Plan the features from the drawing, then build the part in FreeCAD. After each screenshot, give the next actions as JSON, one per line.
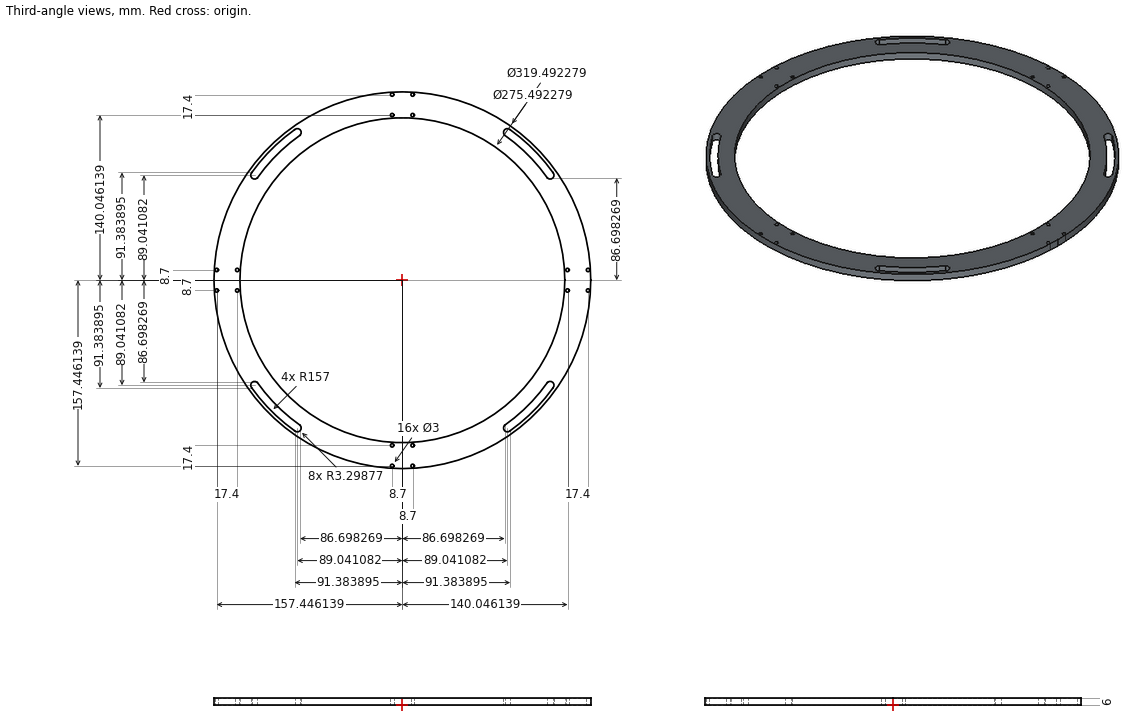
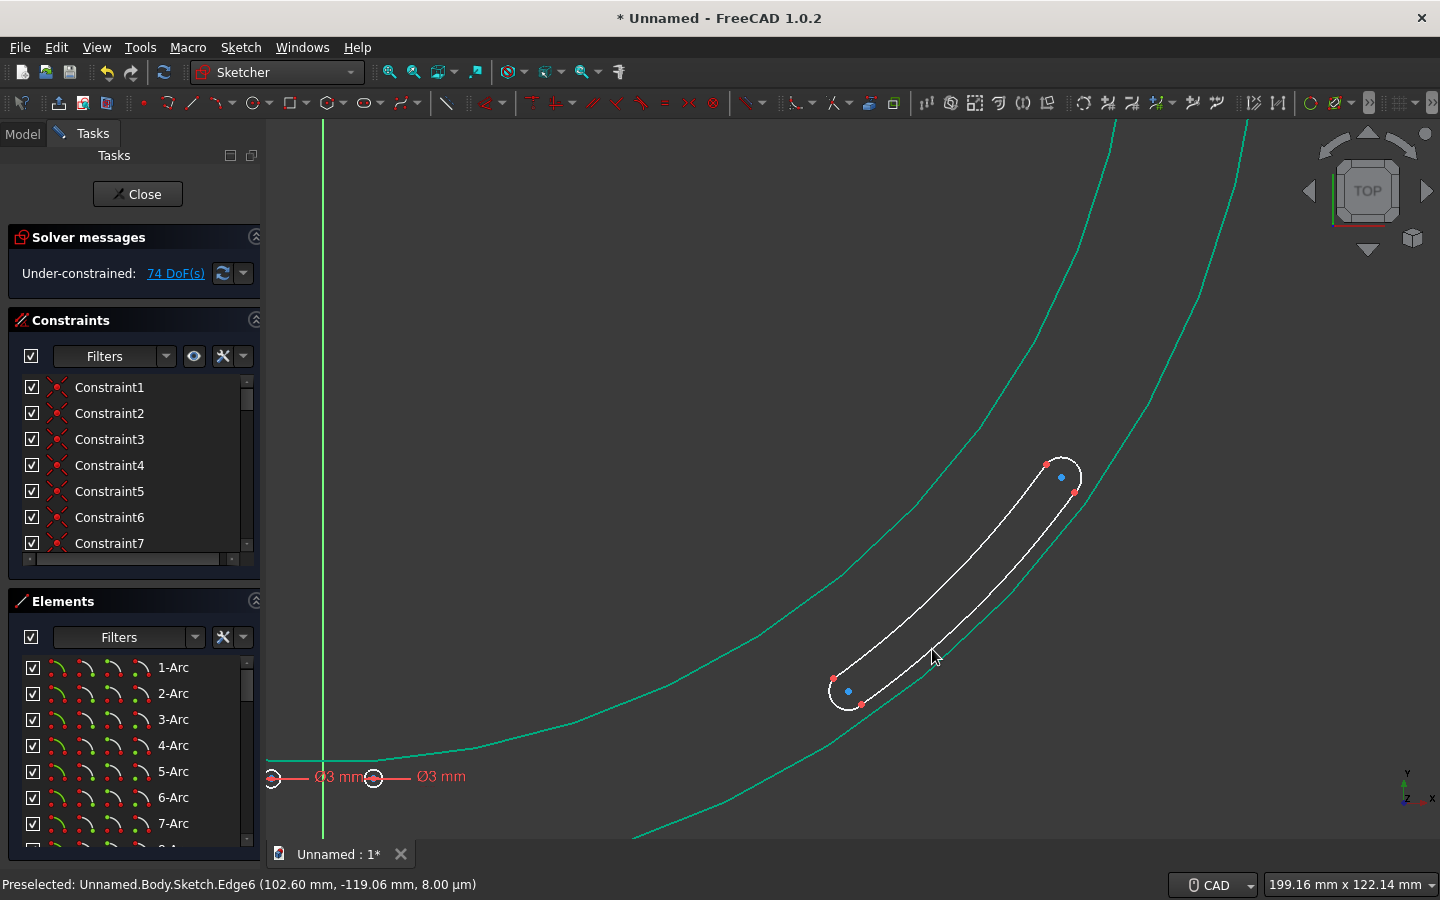
{"action": "left_click", "coordinate": [991, 614]}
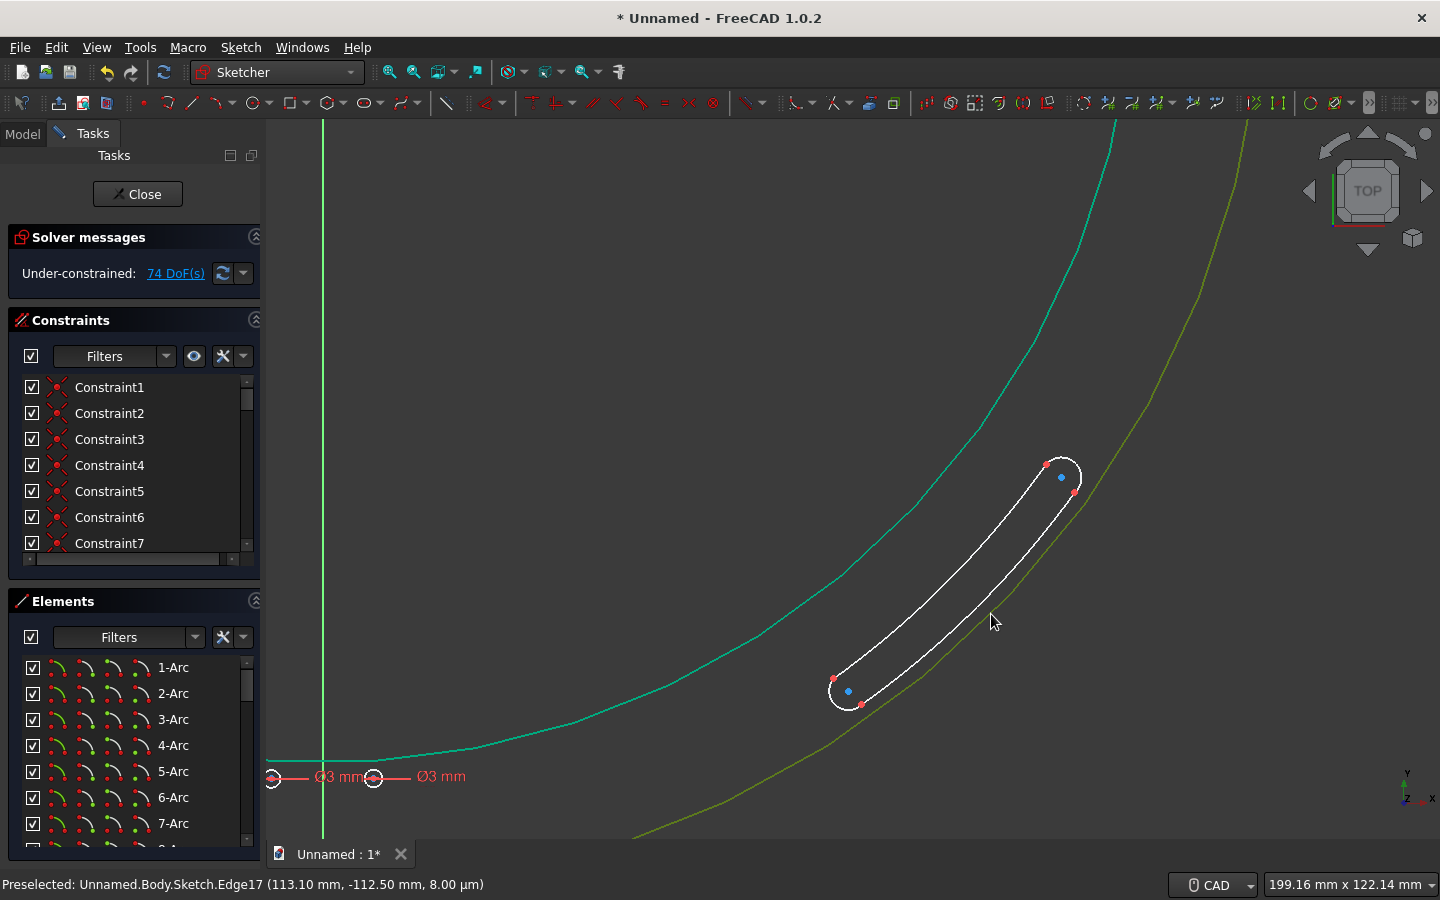
{"action": "left_click", "coordinate": [905, 622]}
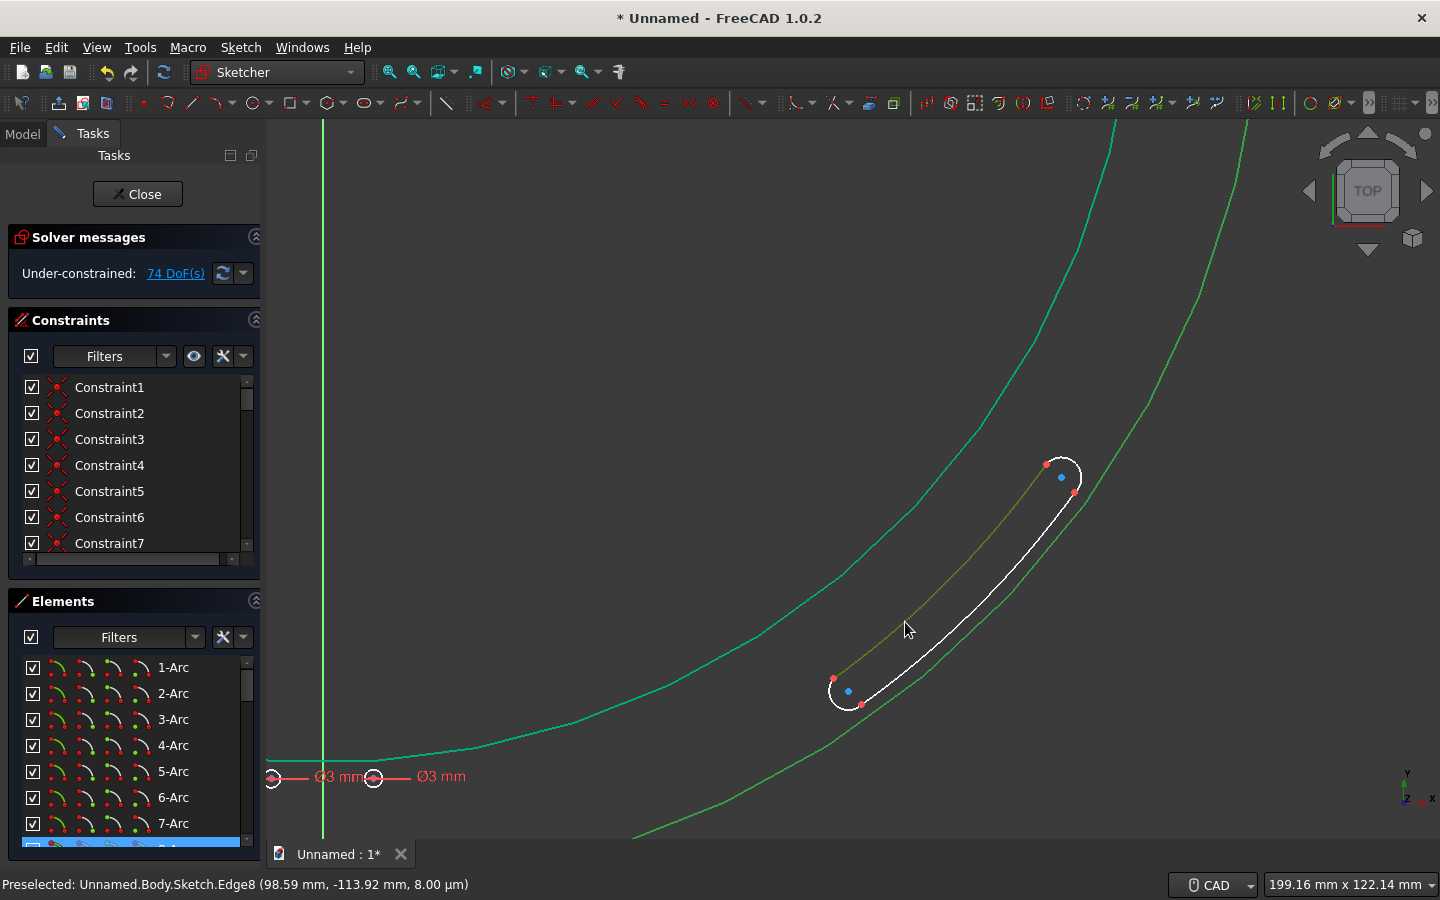
{"action": "left_click", "coordinate": [532, 104]}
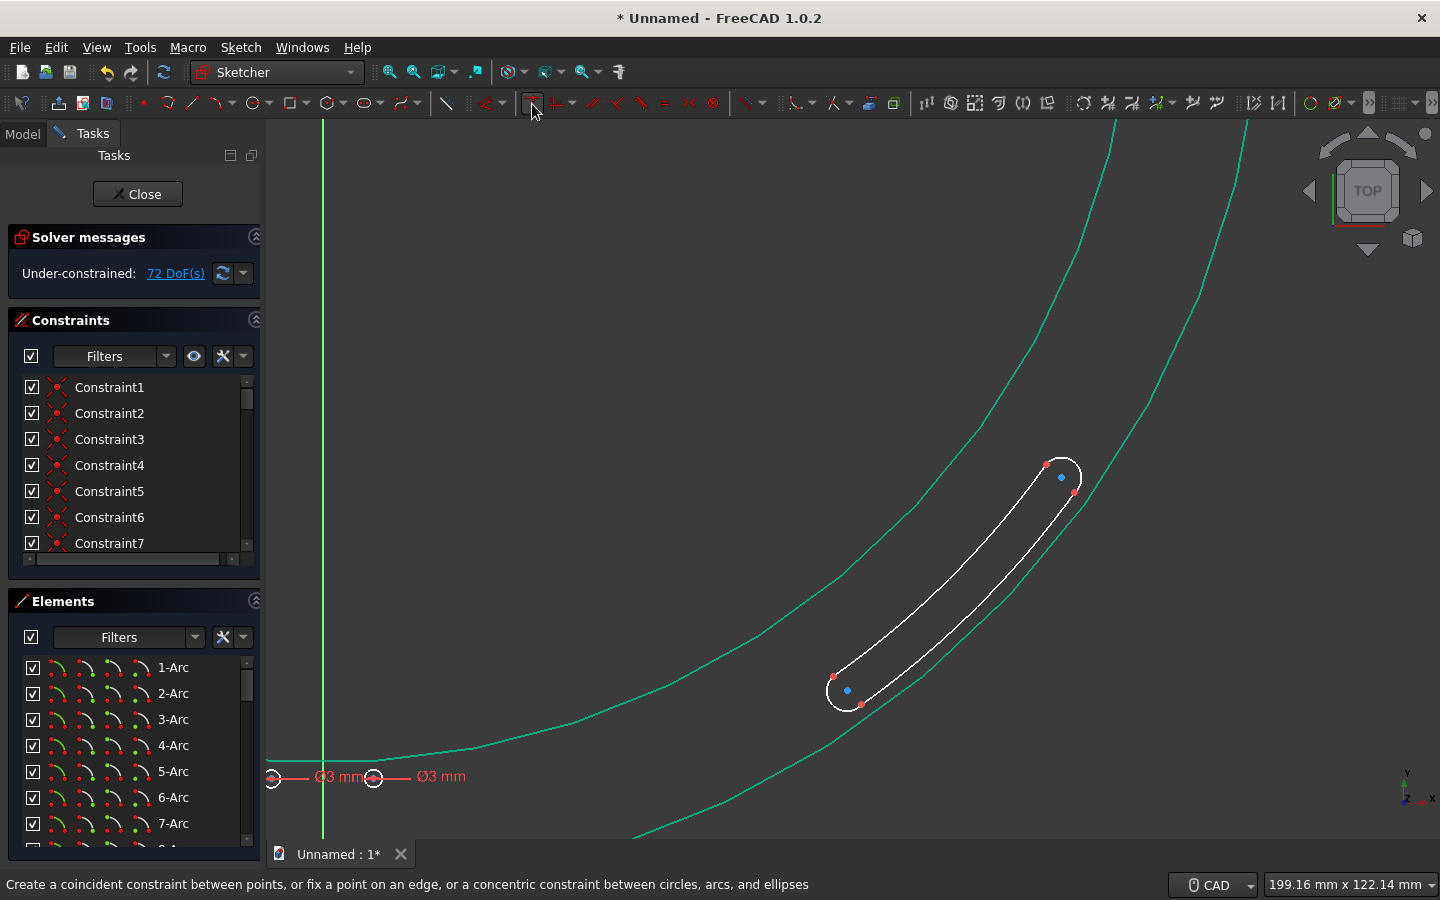
{"action": "left_click", "coordinate": [991, 614]}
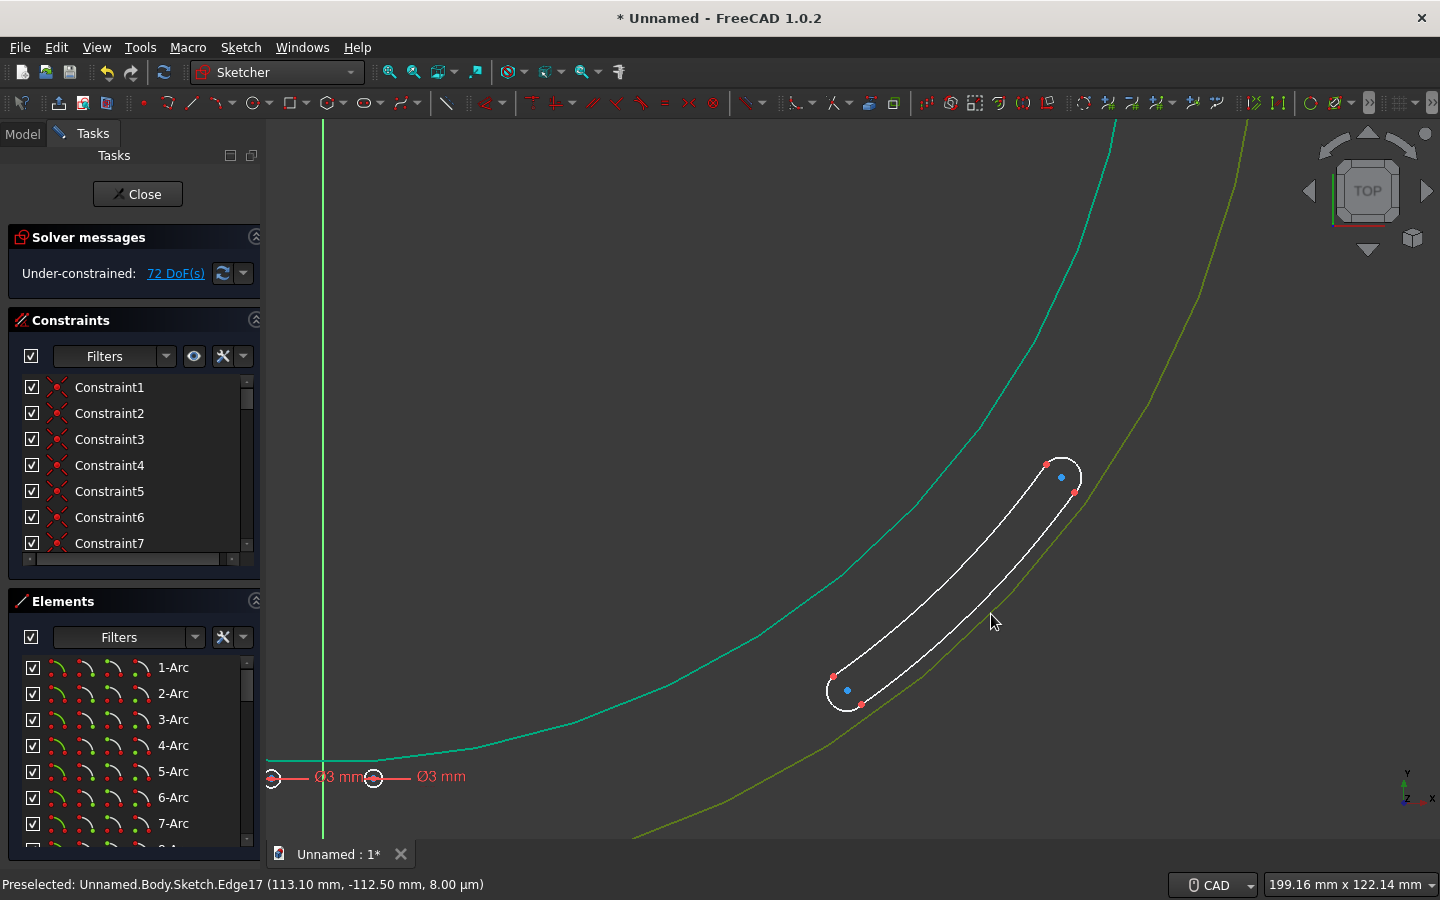
{"action": "scroll", "coordinate": [936, 652], "scroll_direction": "down", "scroll_amount": 7}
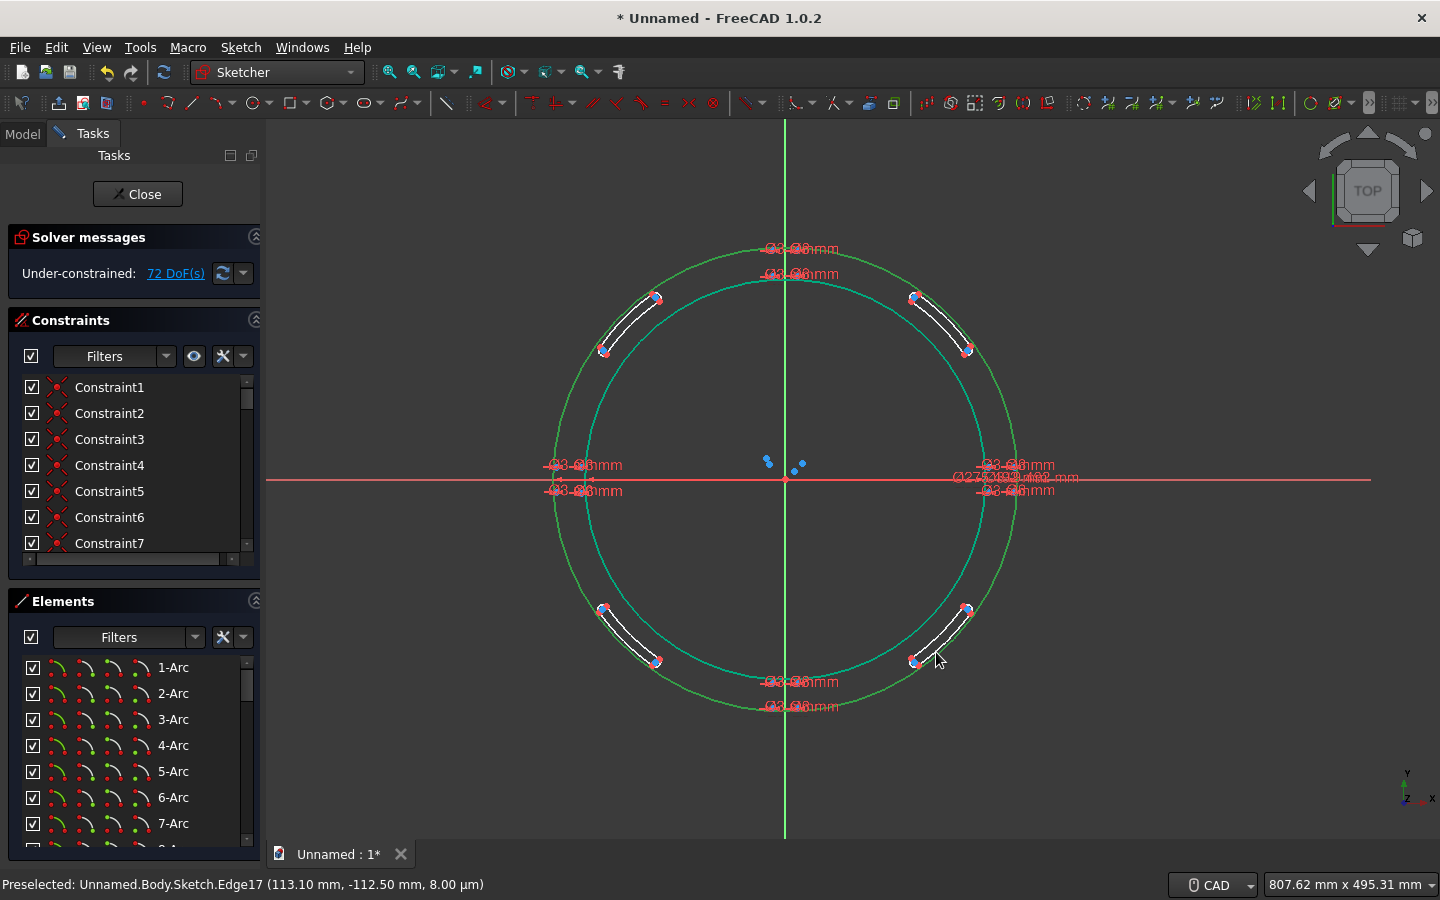
{"action": "scroll", "coordinate": [635, 308], "scroll_direction": "up", "scroll_amount": 7}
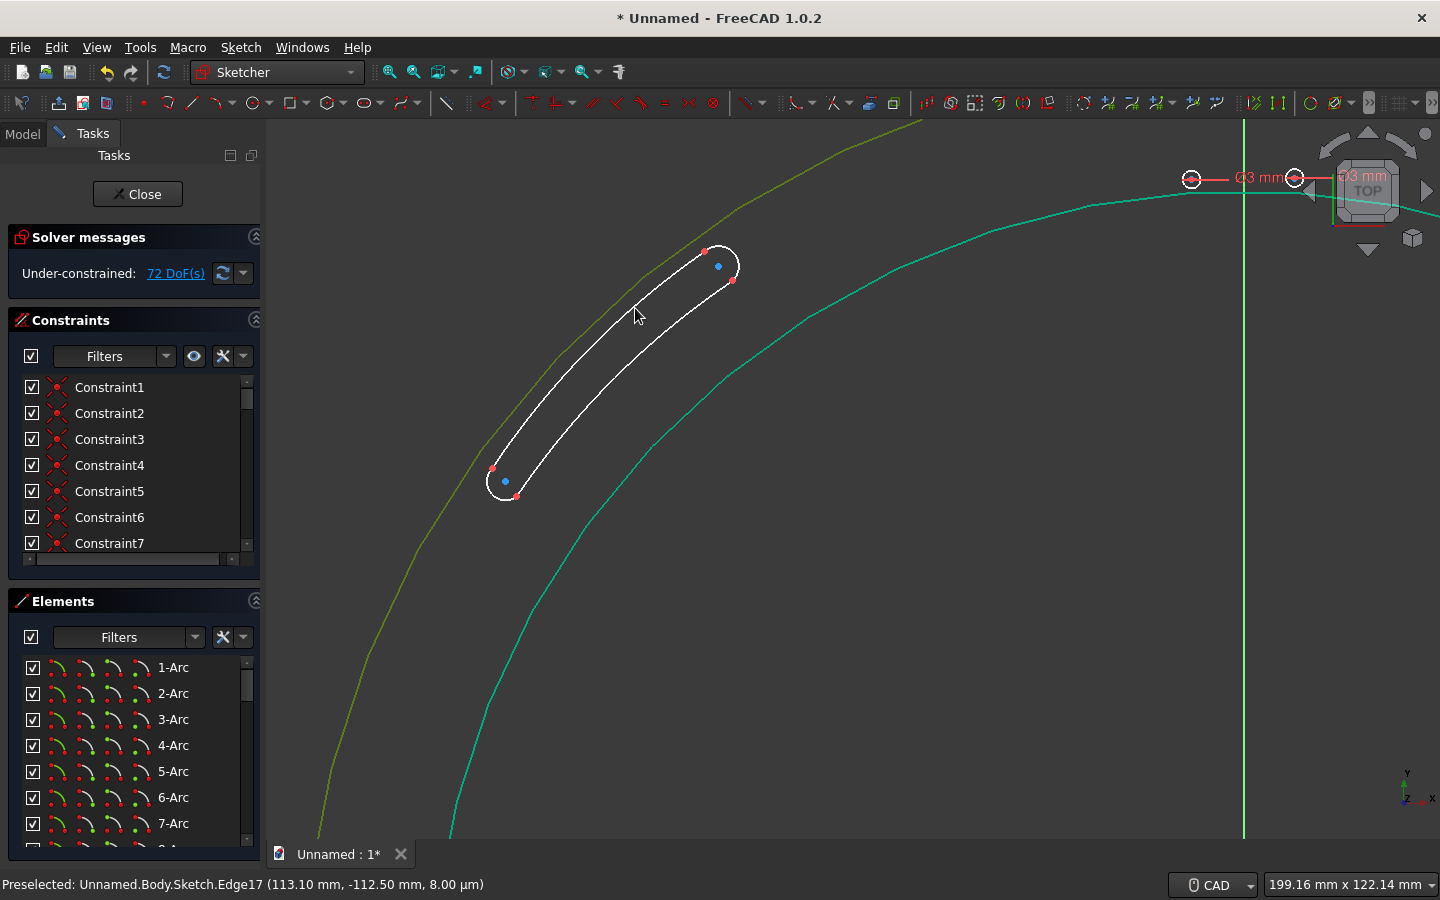
{"action": "left_click", "coordinate": [632, 308]}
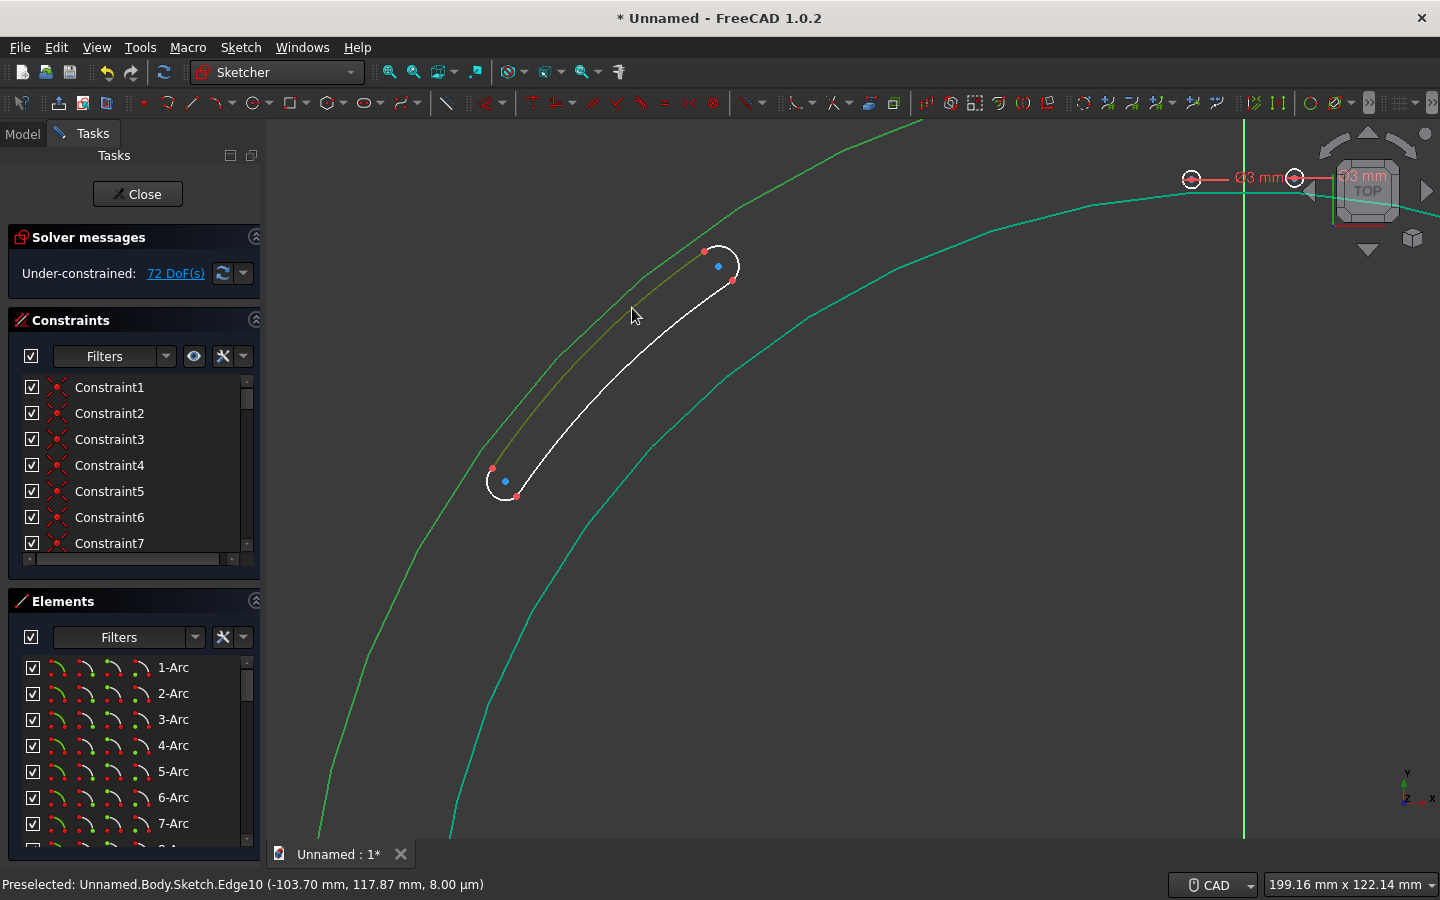
{"action": "key", "text": "c"}